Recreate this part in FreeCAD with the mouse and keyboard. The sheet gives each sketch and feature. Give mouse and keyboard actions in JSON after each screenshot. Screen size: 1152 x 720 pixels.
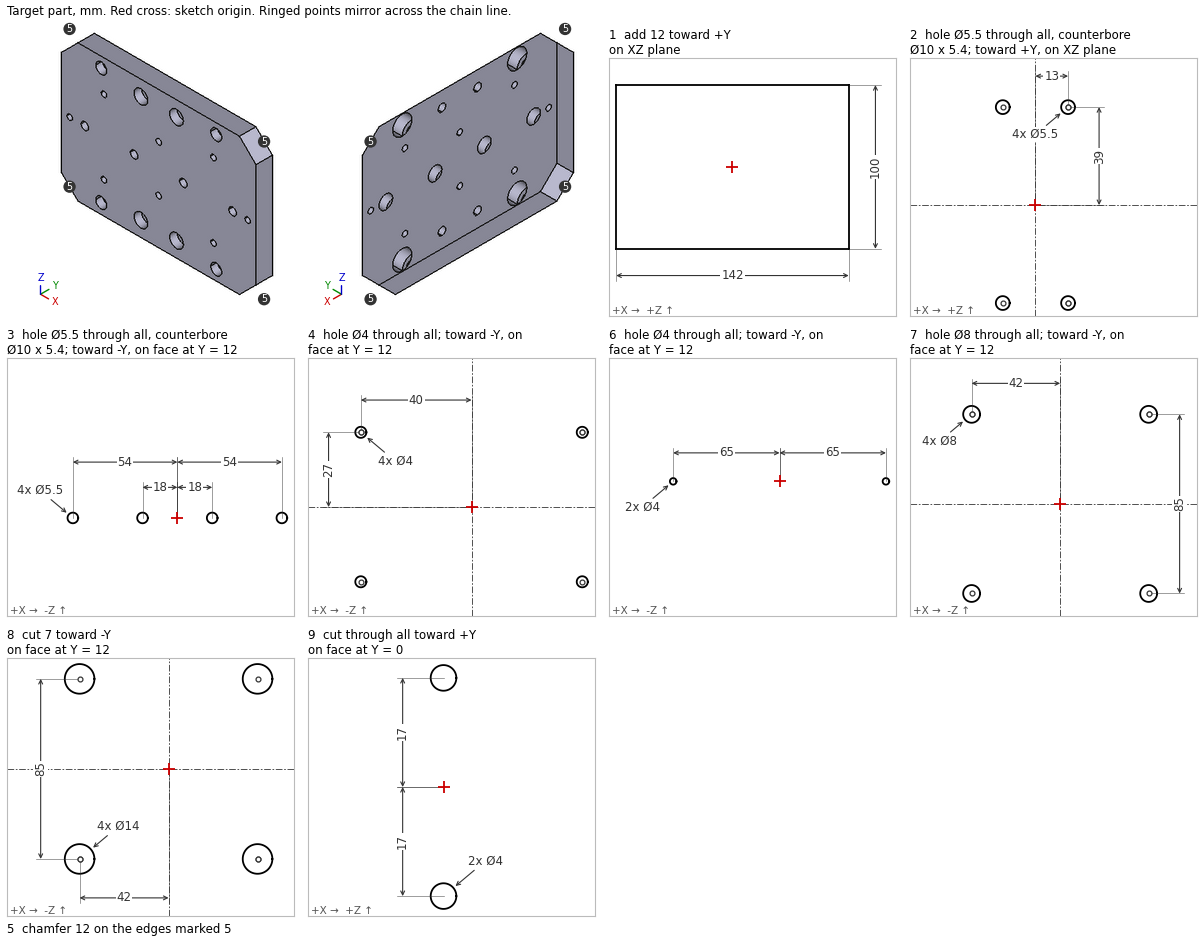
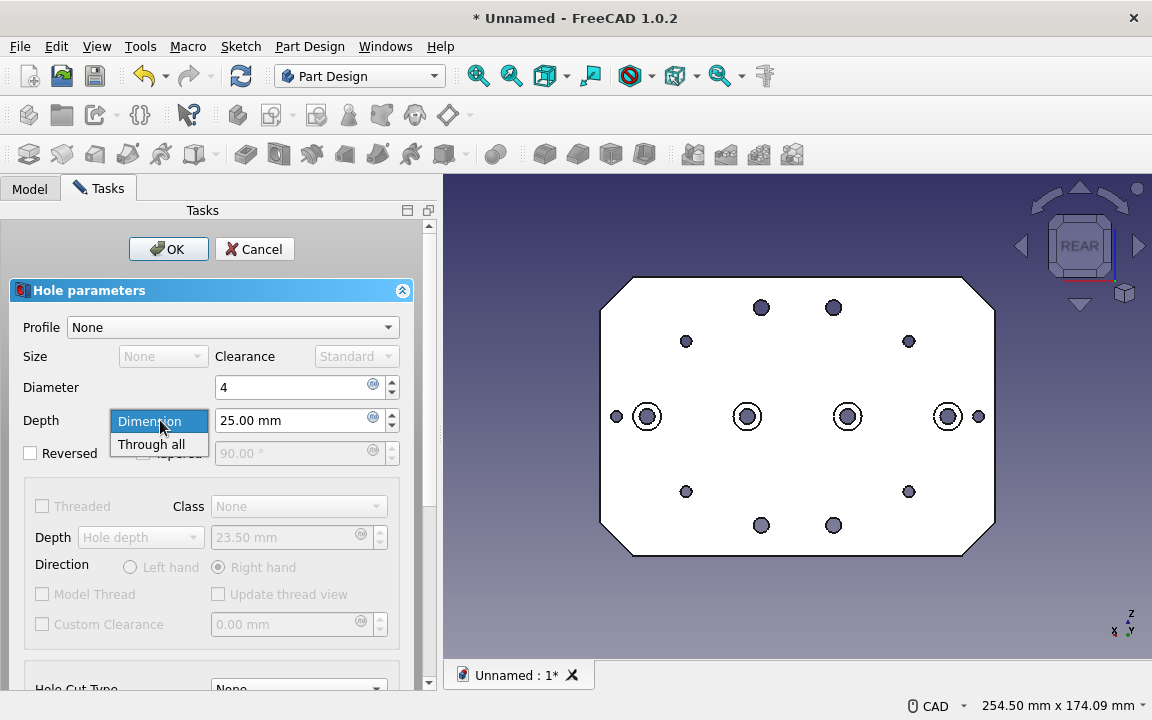
{"action": "left_click", "coordinate": [158, 444]}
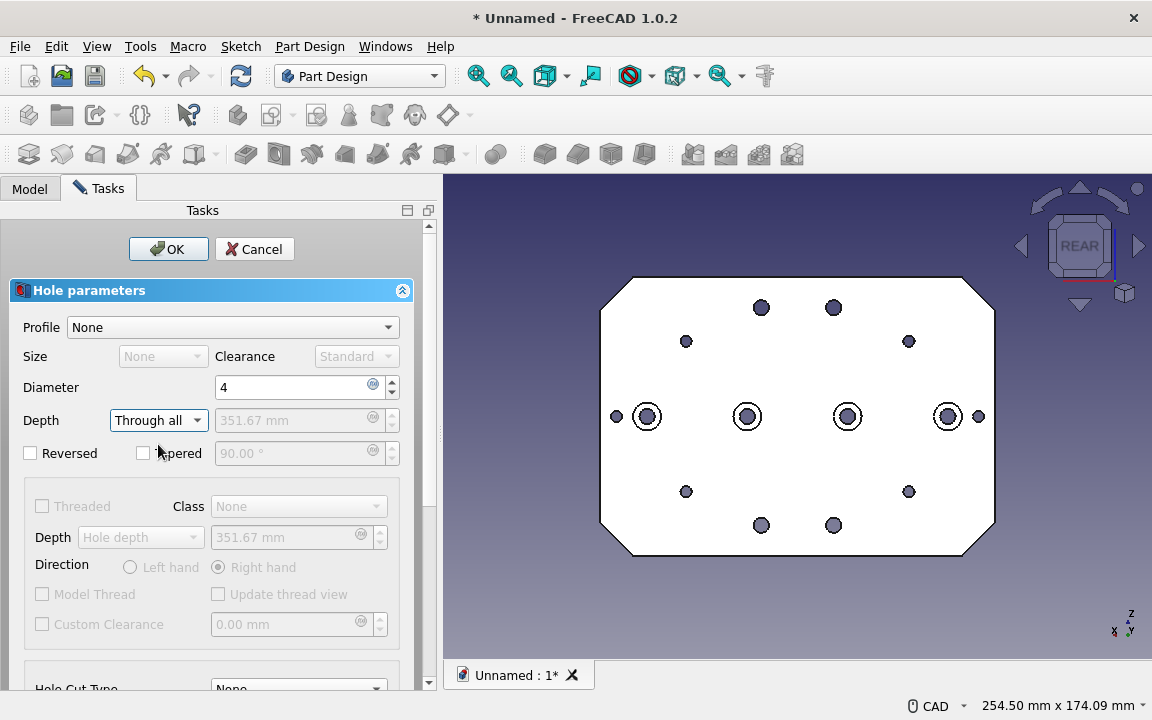
{"action": "left_click", "coordinate": [169, 249]}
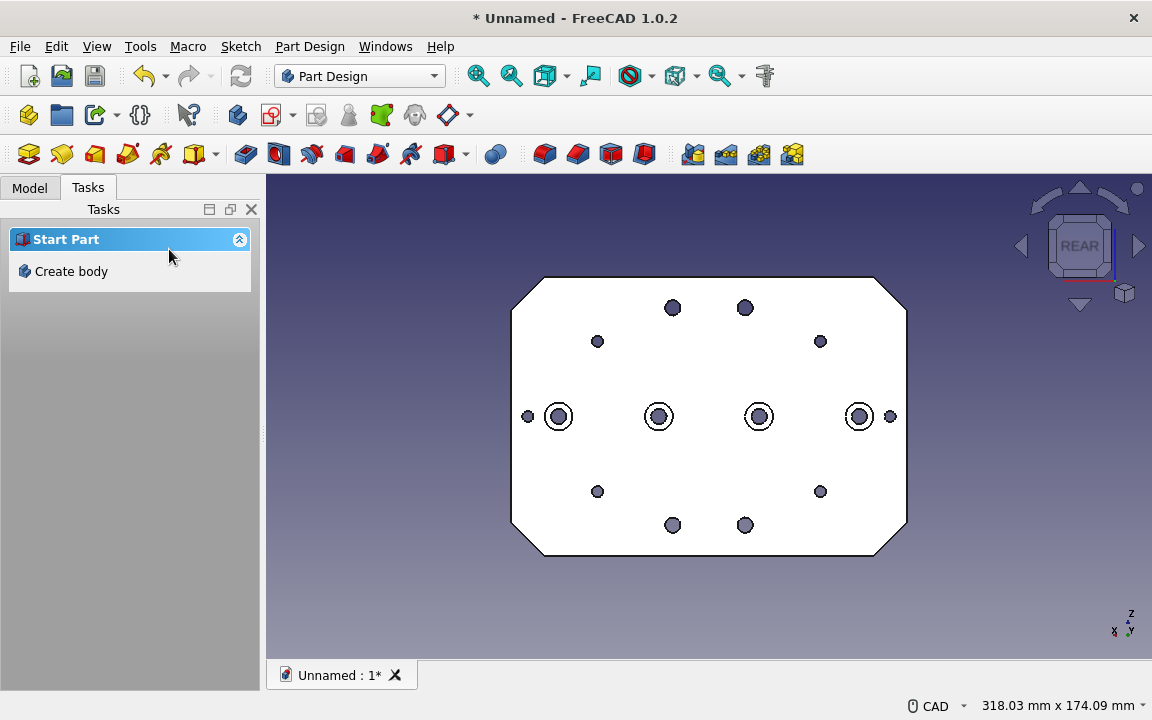
{"action": "left_click", "coordinate": [709, 455]}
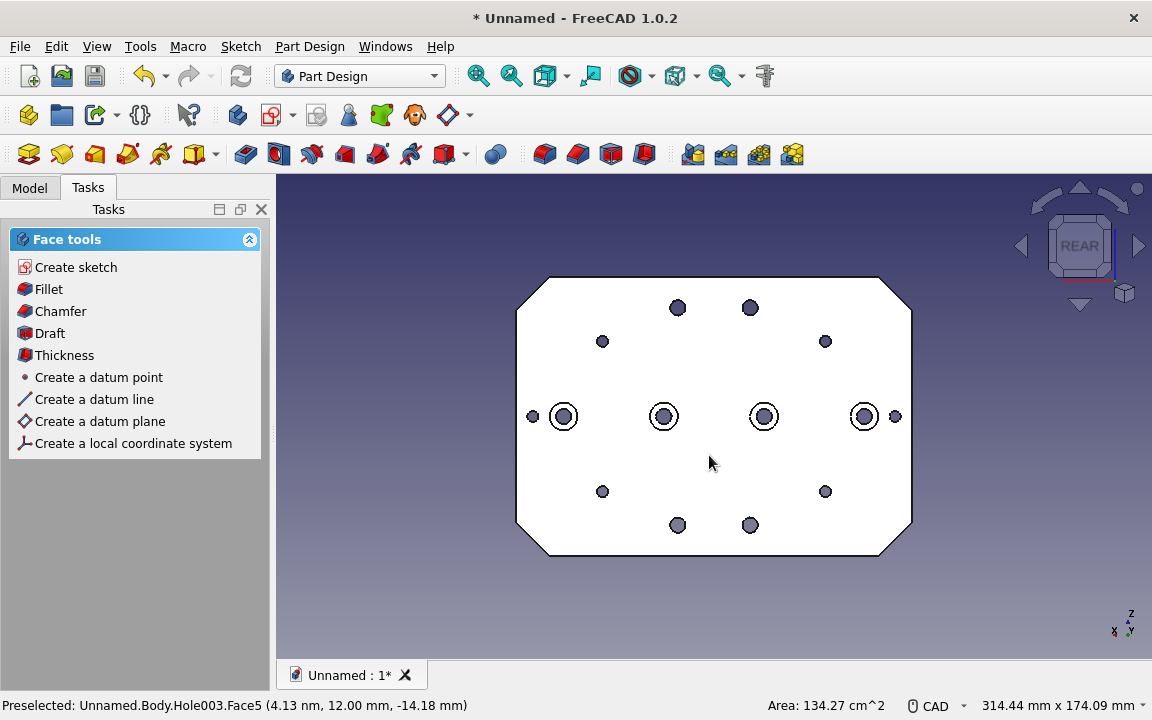
{"action": "left_click", "coordinate": [270, 116]}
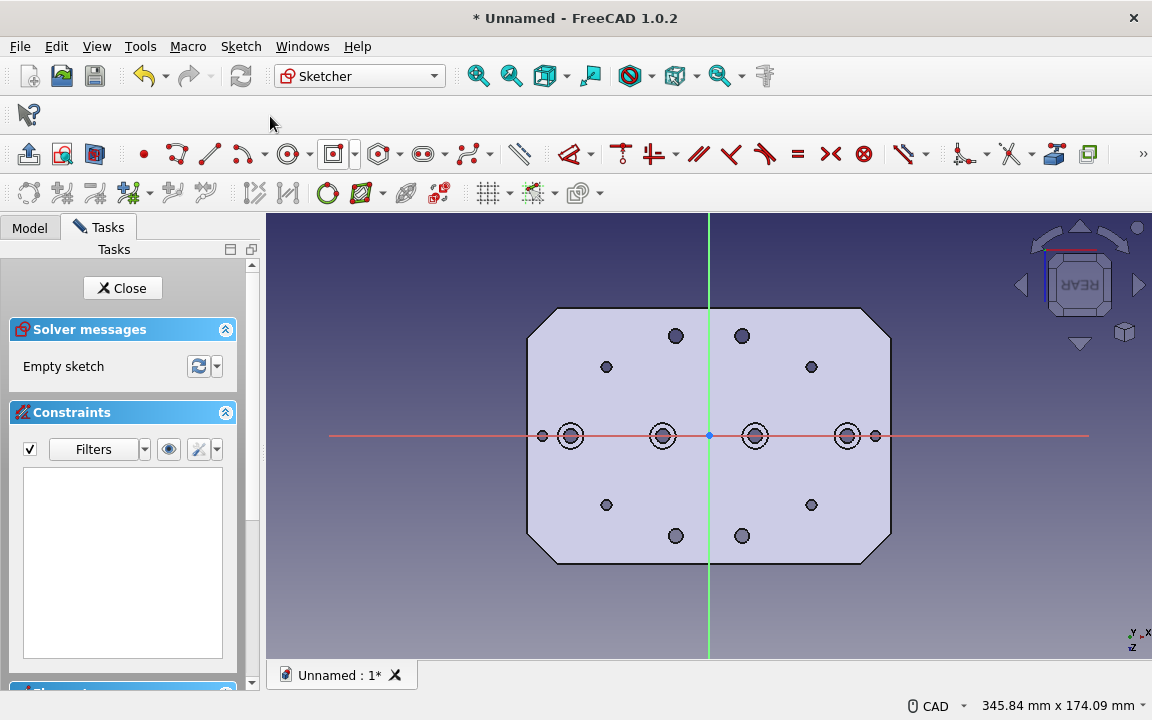
{"action": "left_click", "coordinate": [288, 154]}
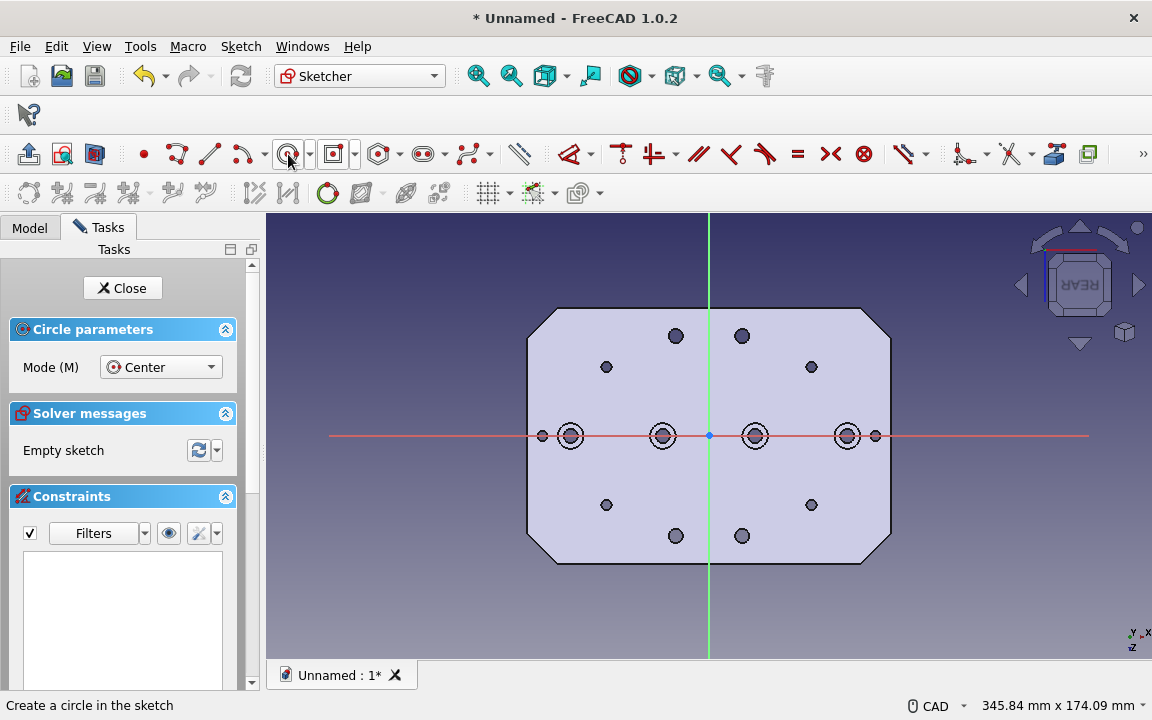
{"action": "scroll", "coordinate": [601, 327], "scroll_direction": "up", "scroll_amount": 4}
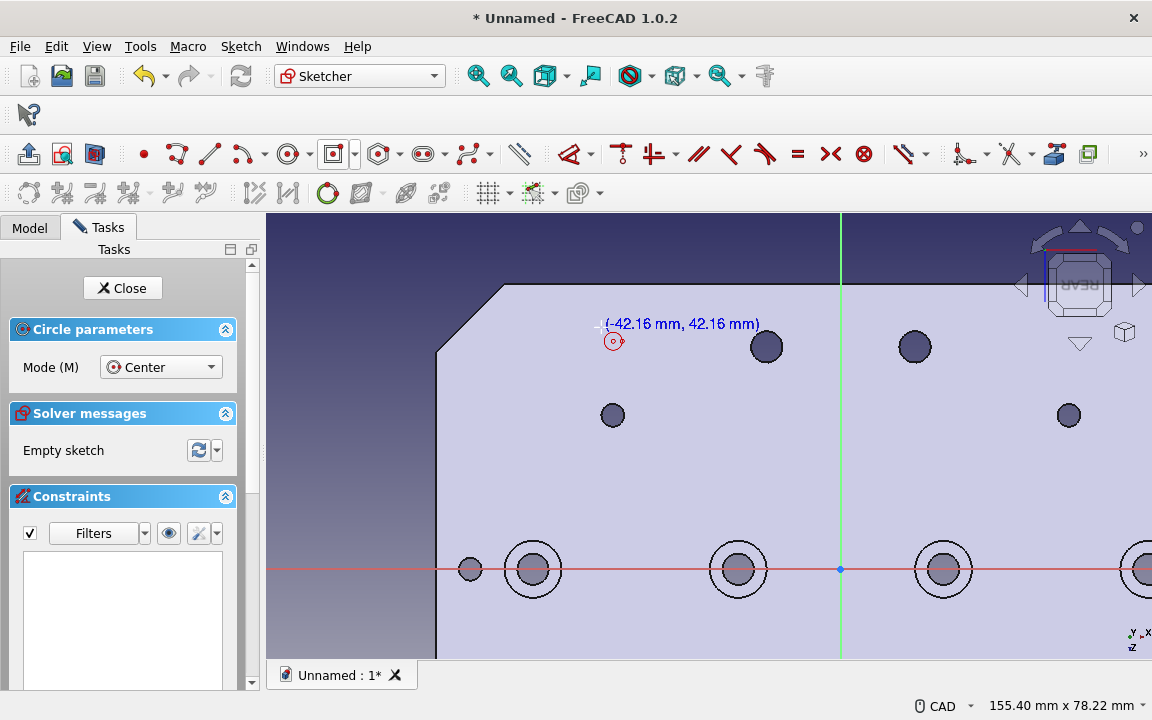
{"action": "left_click", "coordinate": [601, 327]}
{"action": "left_click", "coordinate": [618, 311]}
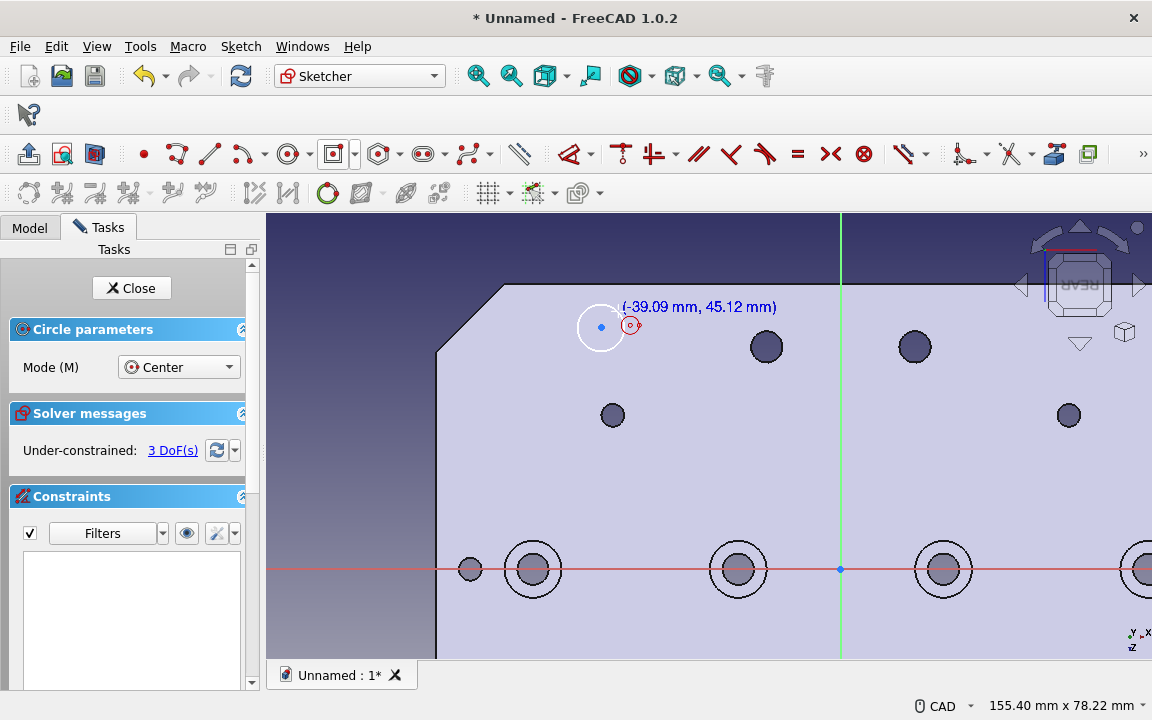
{"action": "scroll", "coordinate": [397, 274], "scroll_direction": "down", "scroll_amount": 3}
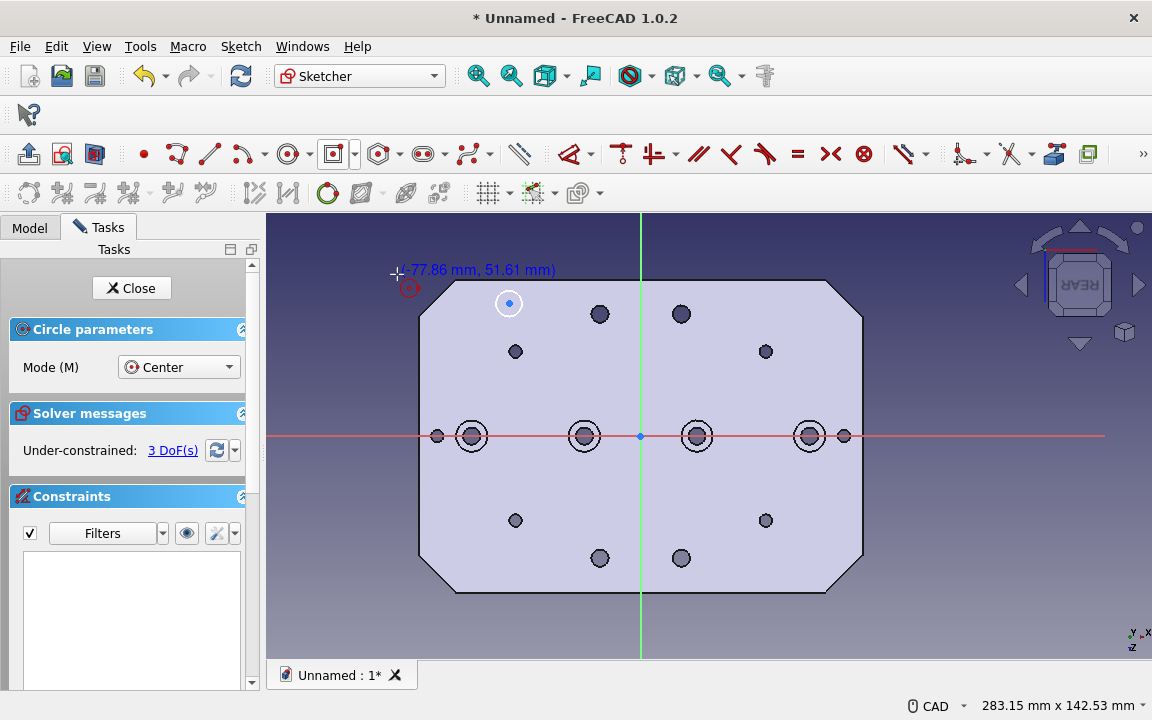
{"action": "scroll", "coordinate": [772, 303], "scroll_direction": "up", "scroll_amount": 3}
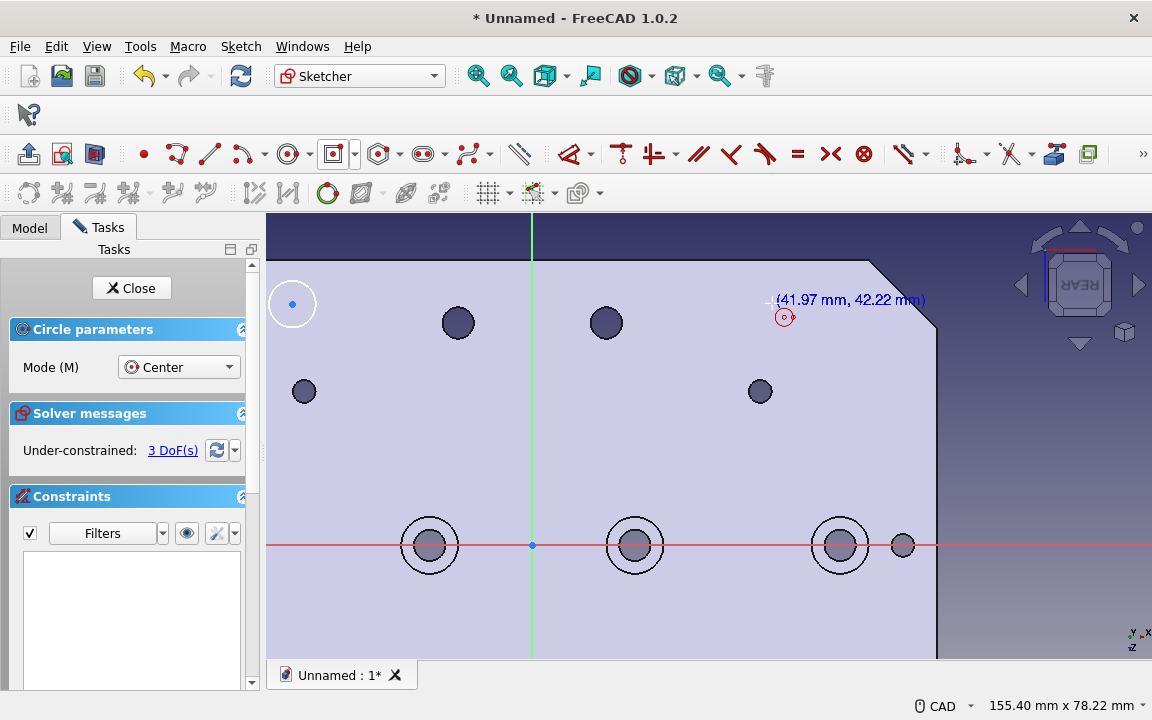
{"action": "left_click", "coordinate": [772, 303]}
{"action": "left_click", "coordinate": [788, 287]}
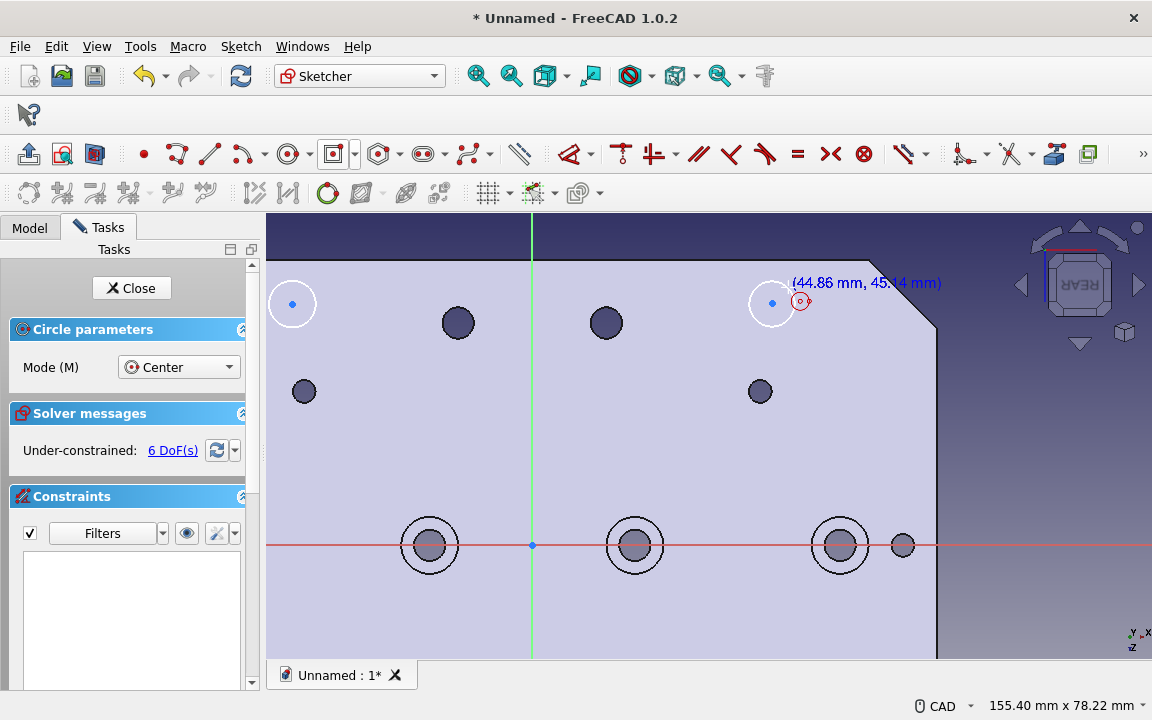
{"action": "scroll", "coordinate": [772, 303], "scroll_direction": "down", "scroll_amount": 3}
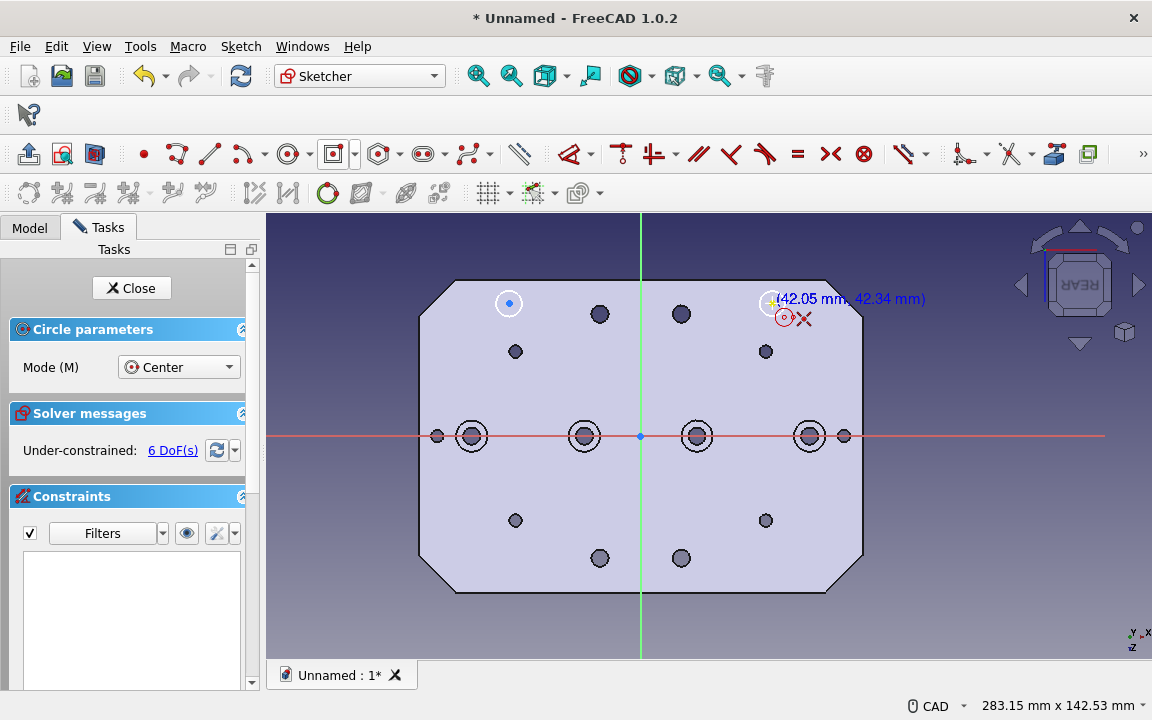
{"action": "scroll", "coordinate": [772, 569], "scroll_direction": "up", "scroll_amount": 3}